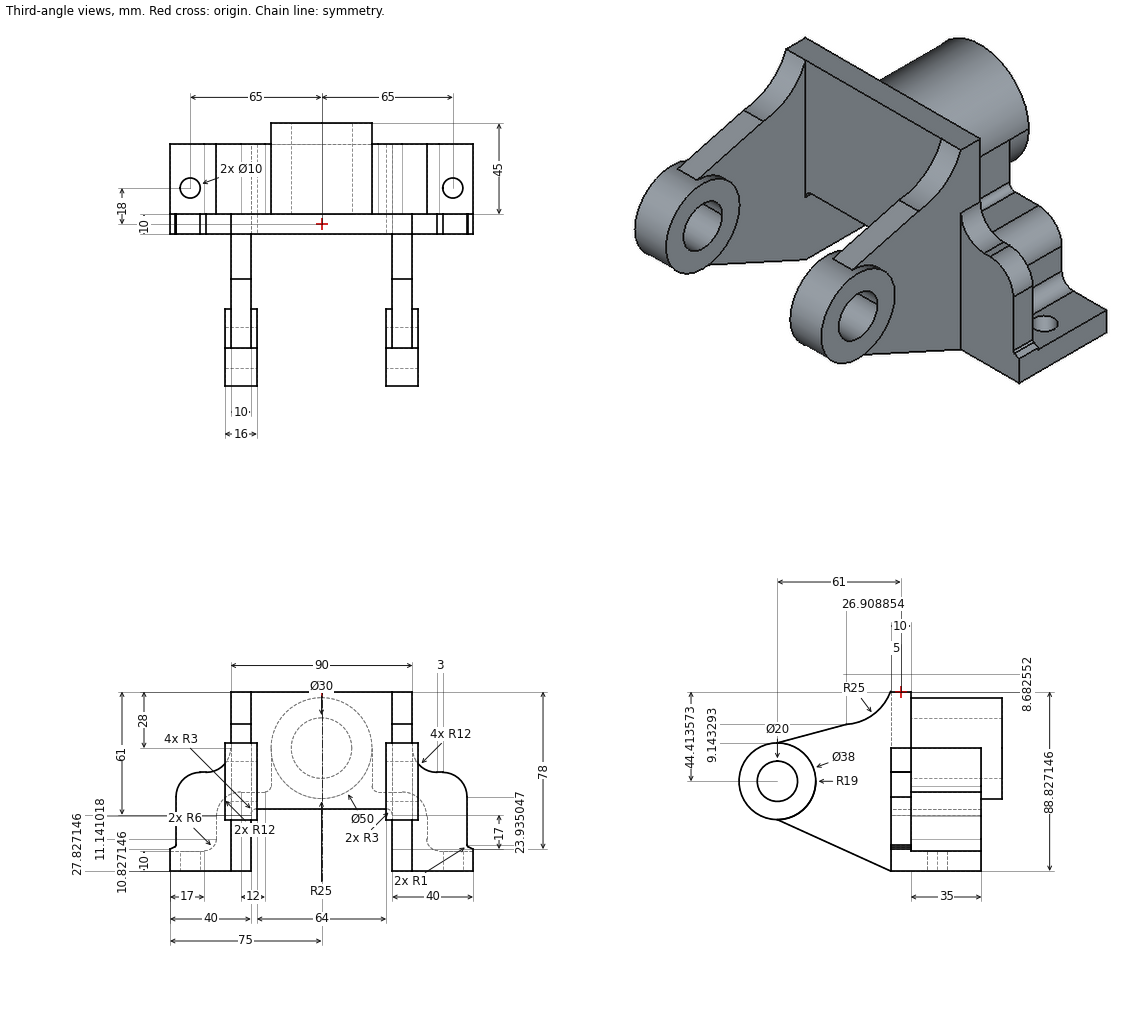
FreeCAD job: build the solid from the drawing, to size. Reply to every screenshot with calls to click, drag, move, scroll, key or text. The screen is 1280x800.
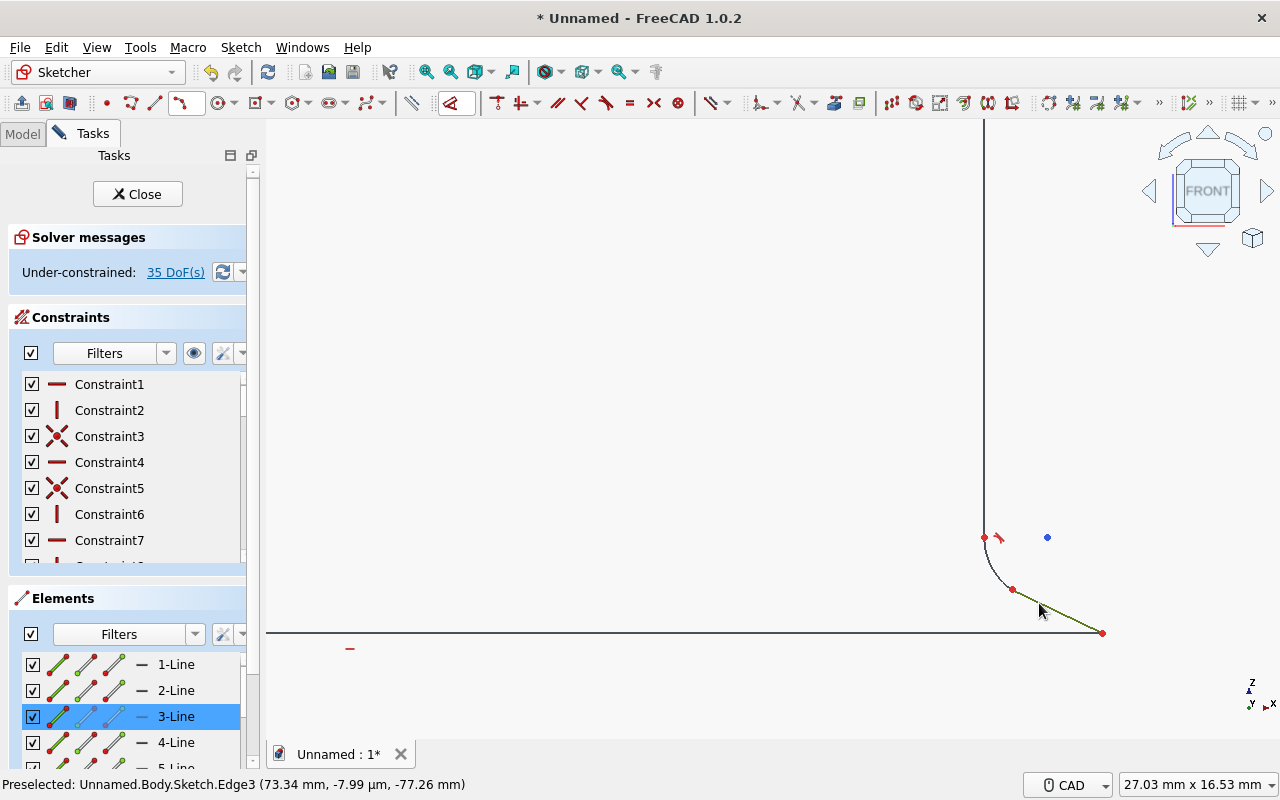
click(987, 556)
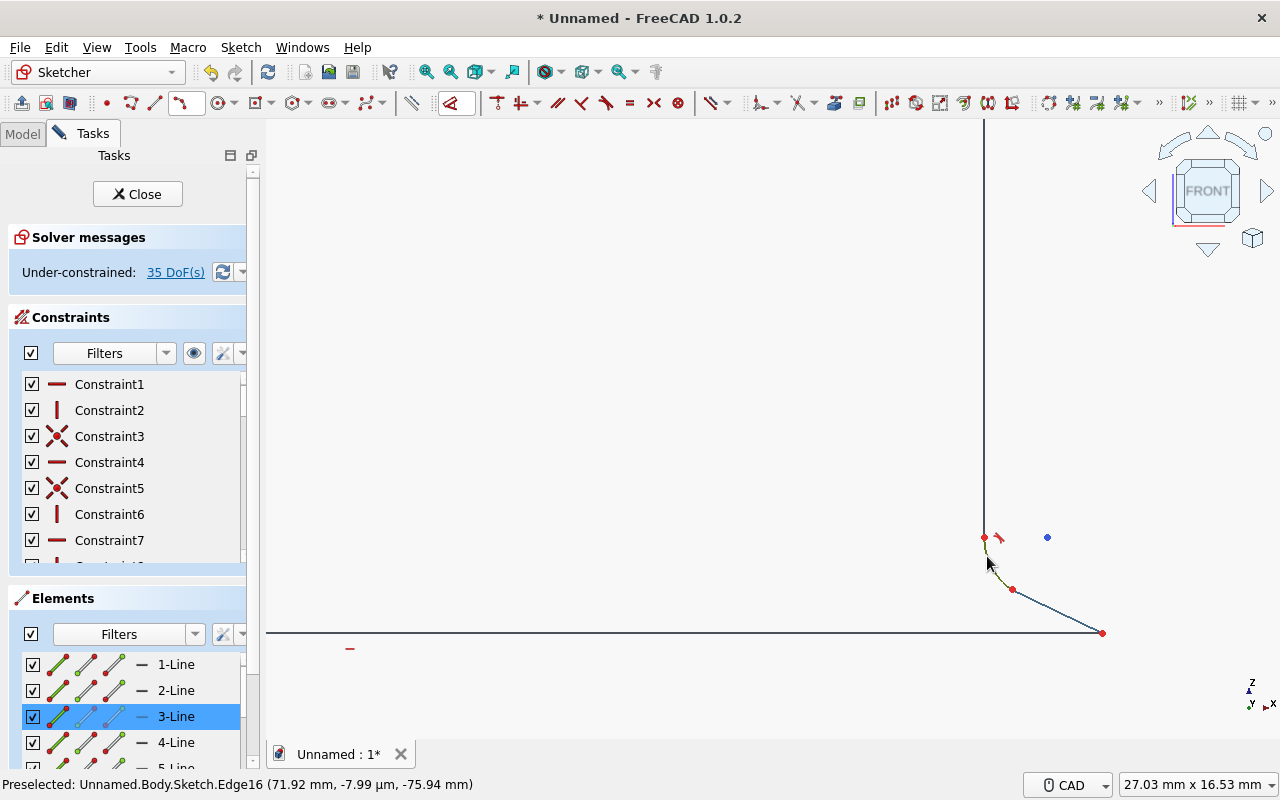
click(606, 104)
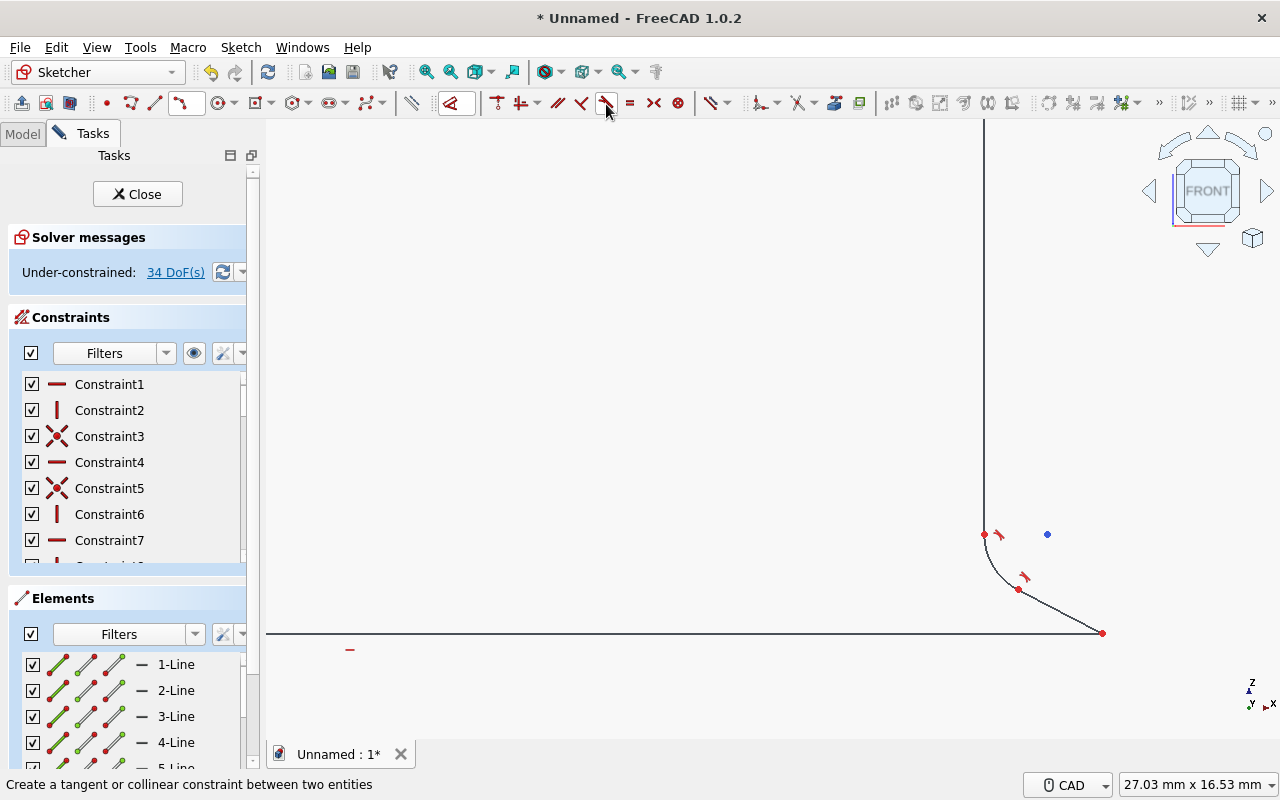
scroll(1006, 586, down, 11)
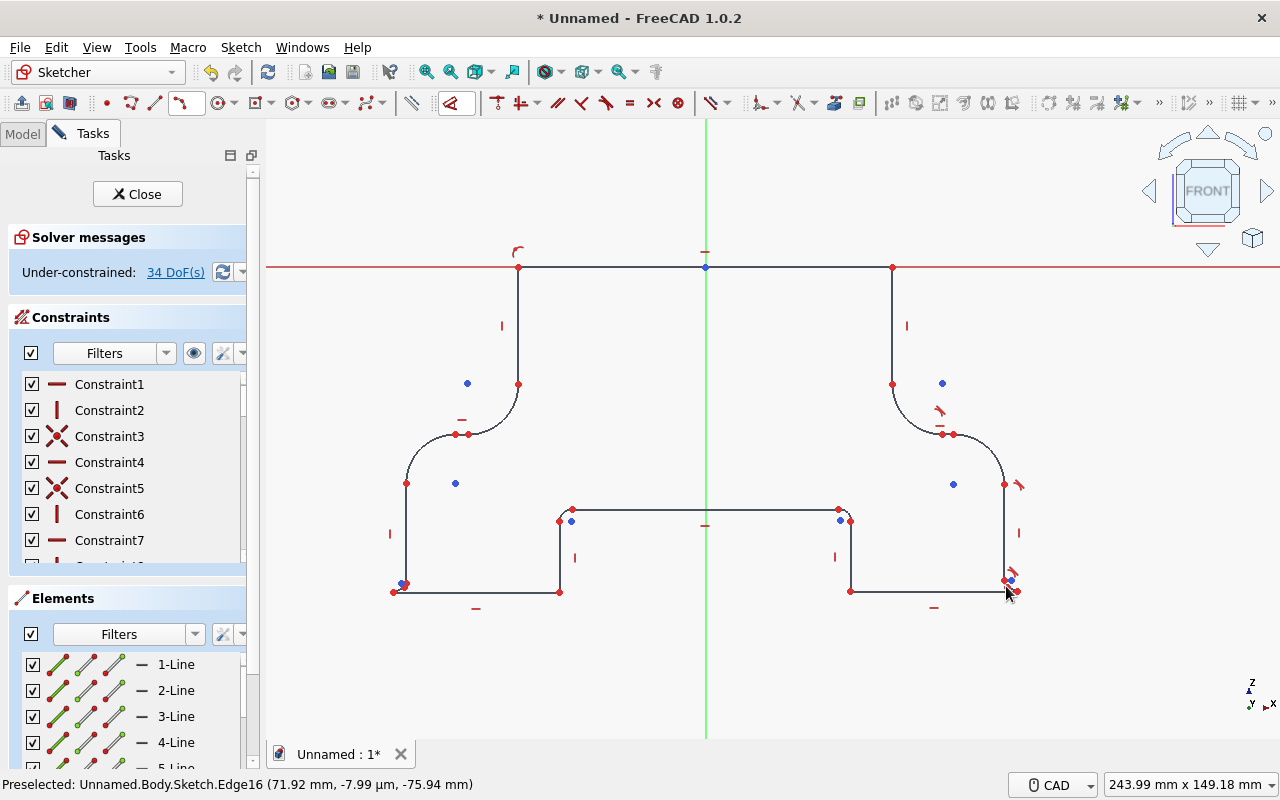
click(851, 571)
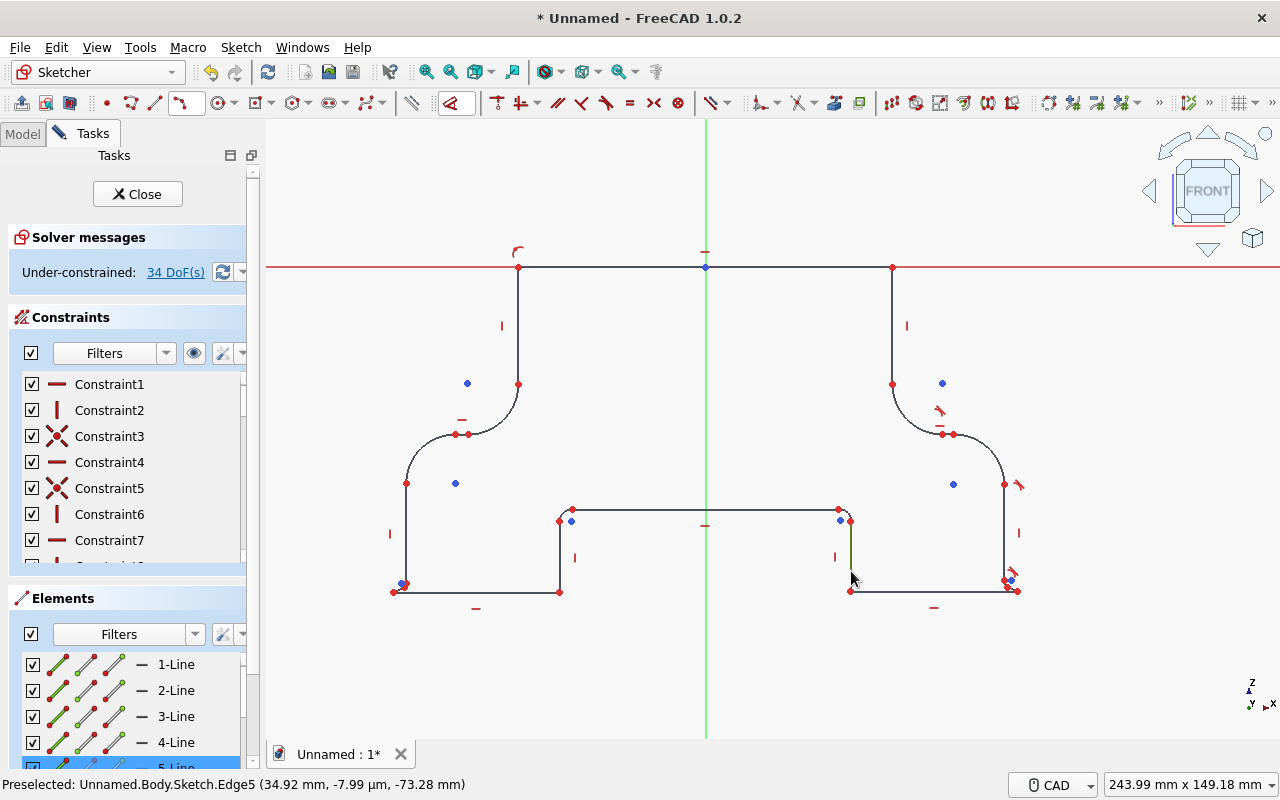
scroll(848, 513, up, 2)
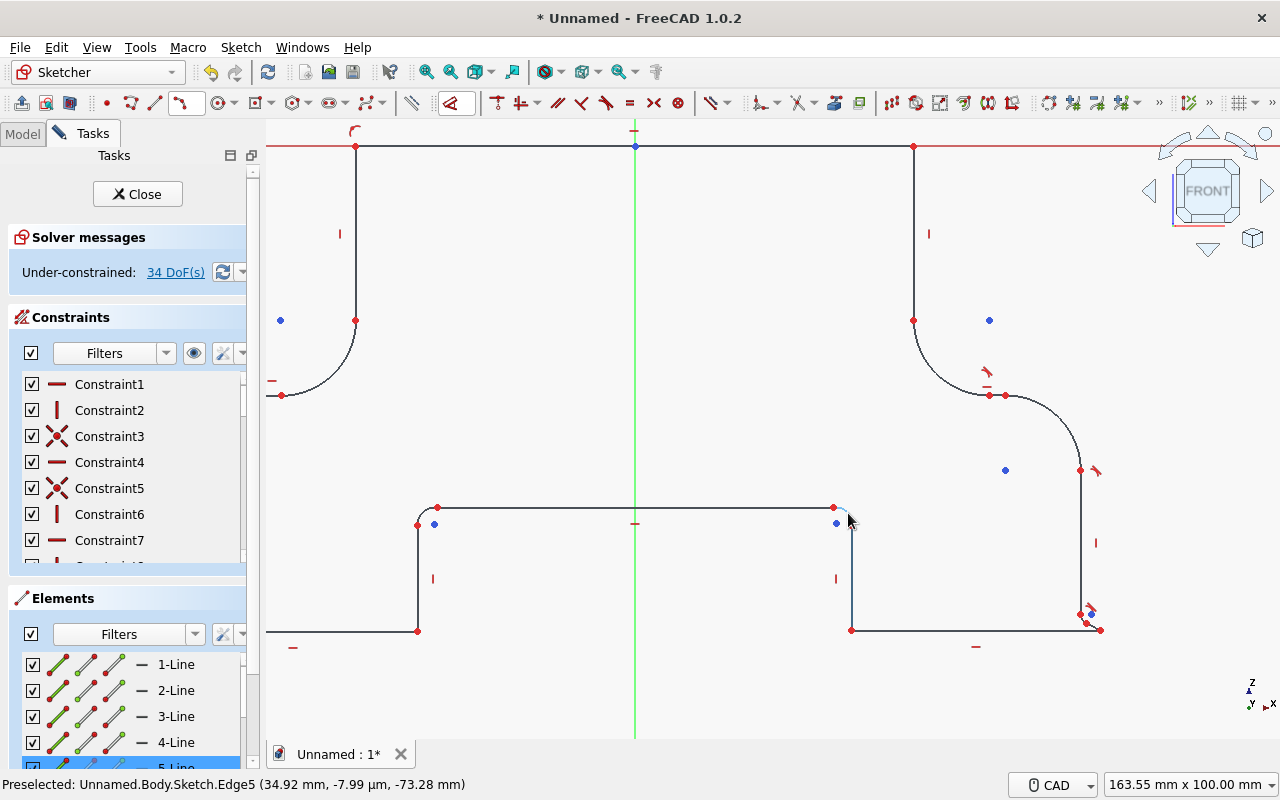
click(847, 512)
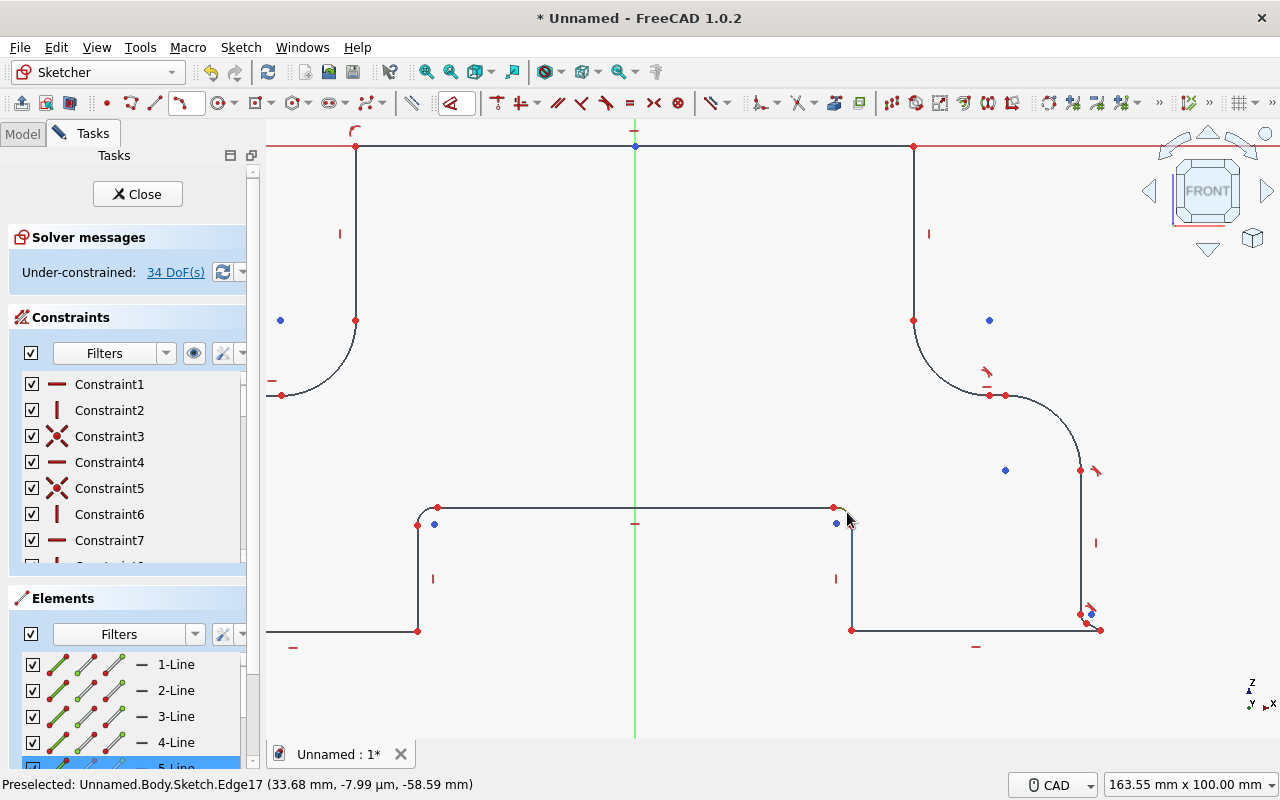
key(t)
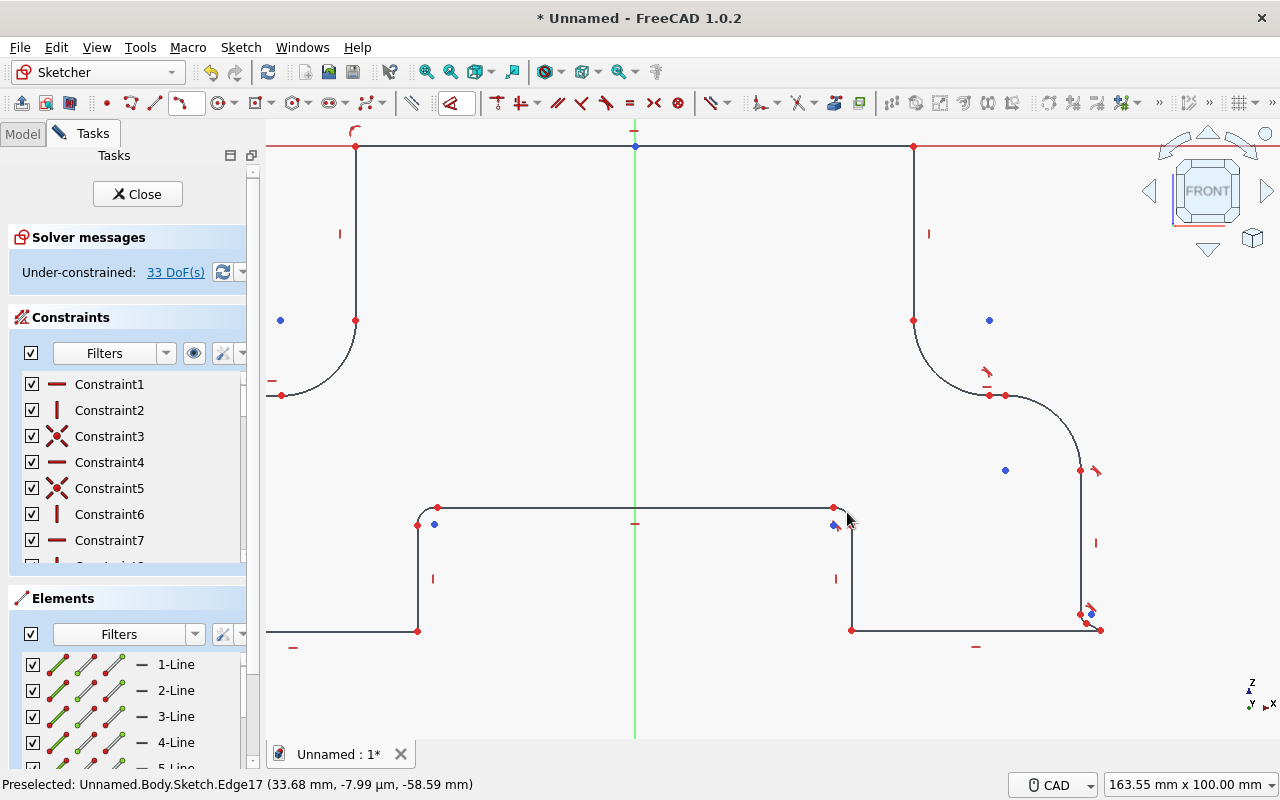
click(715, 508)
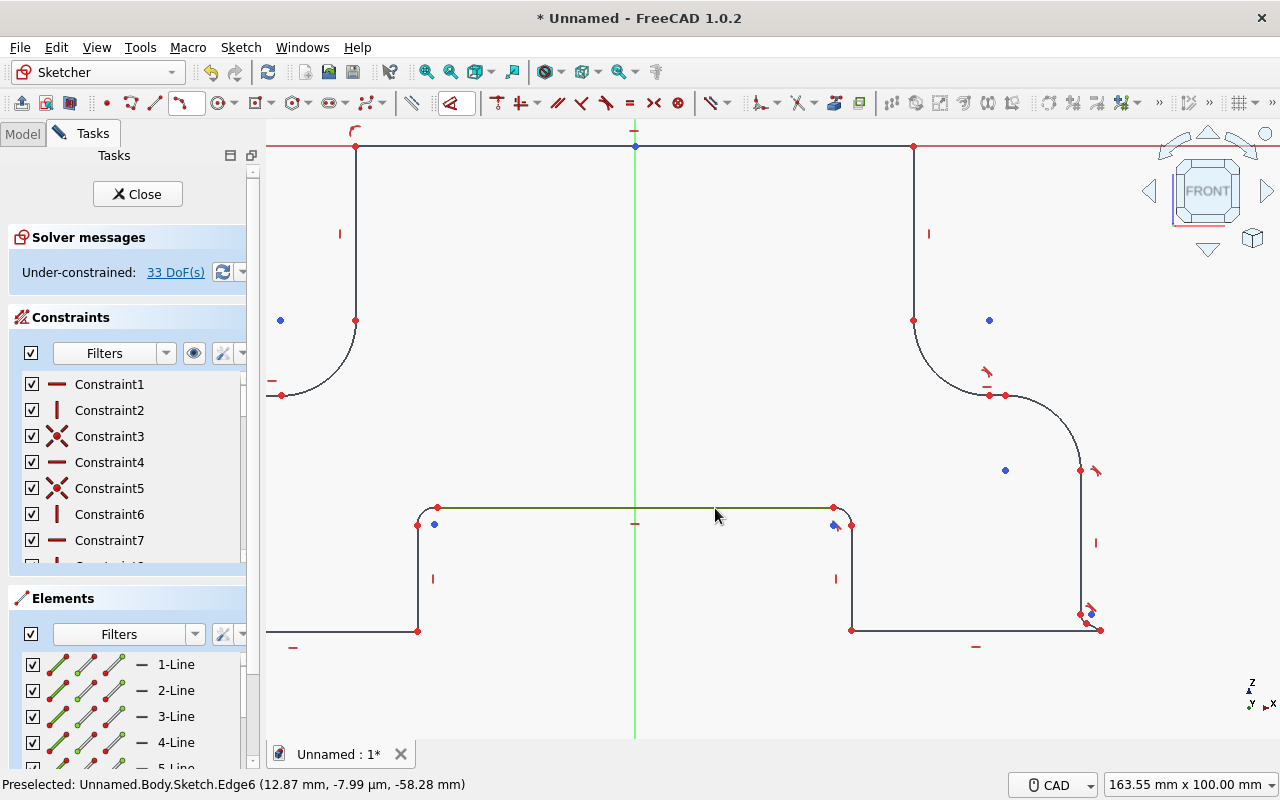
click(847, 513)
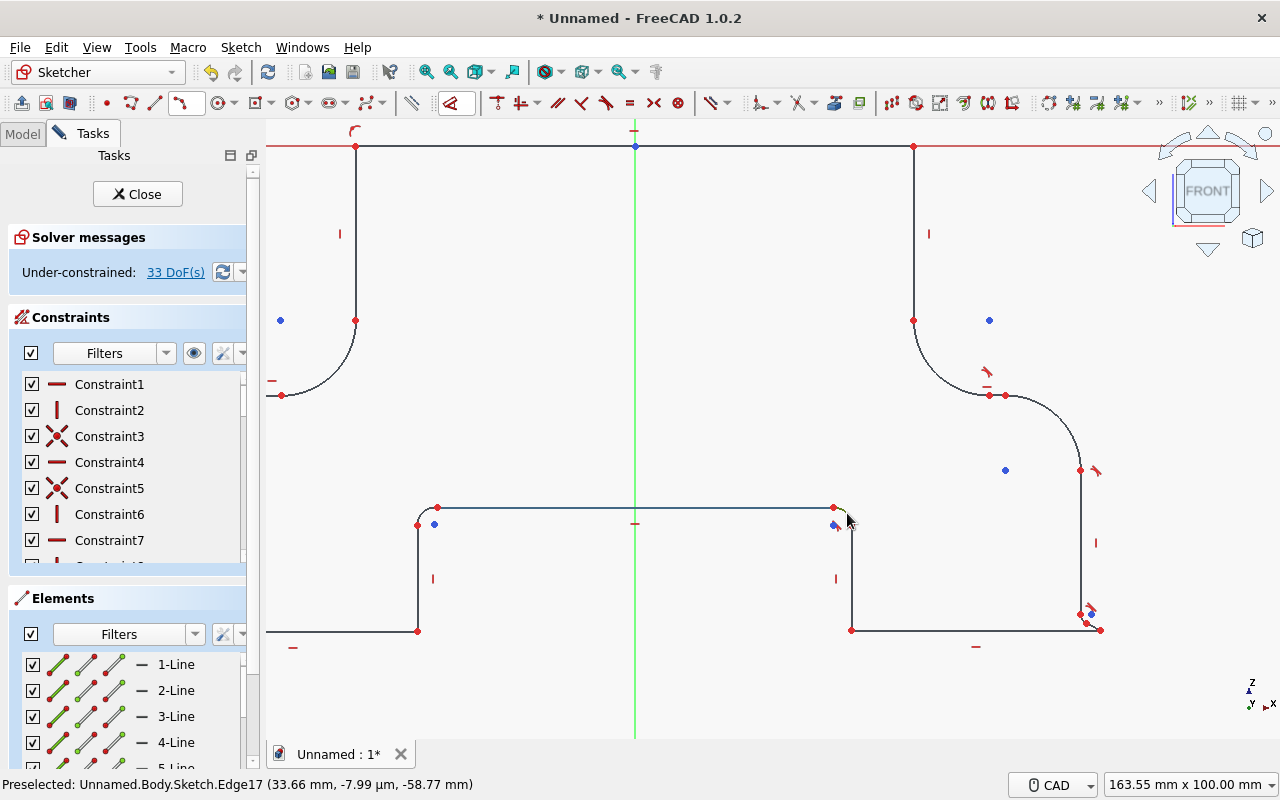
click(606, 104)